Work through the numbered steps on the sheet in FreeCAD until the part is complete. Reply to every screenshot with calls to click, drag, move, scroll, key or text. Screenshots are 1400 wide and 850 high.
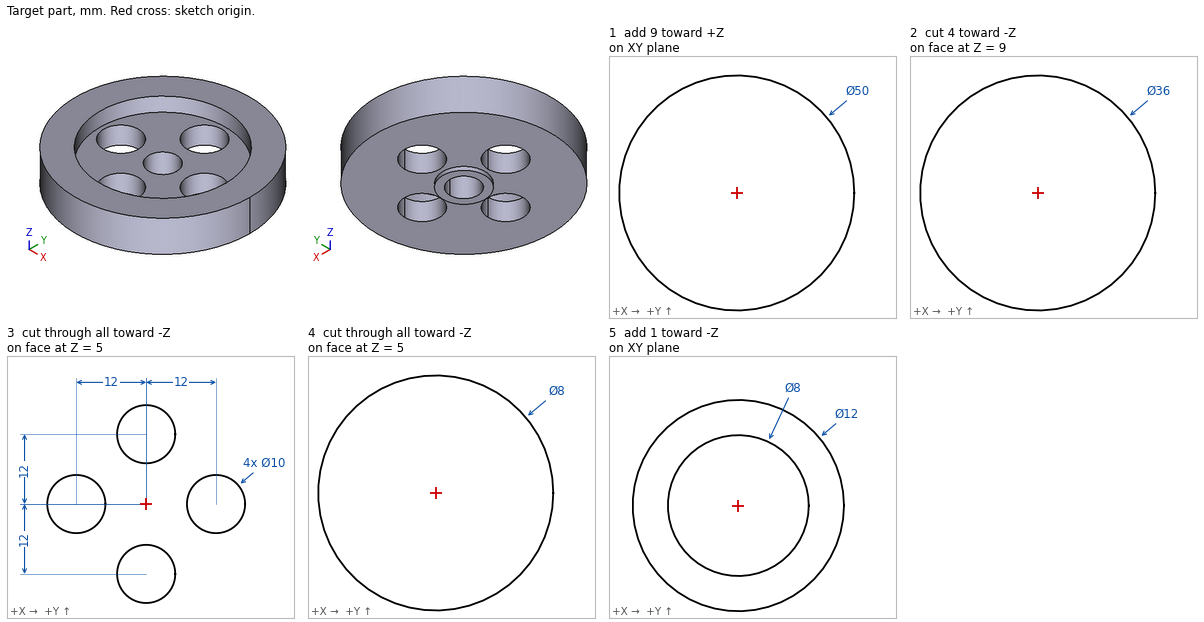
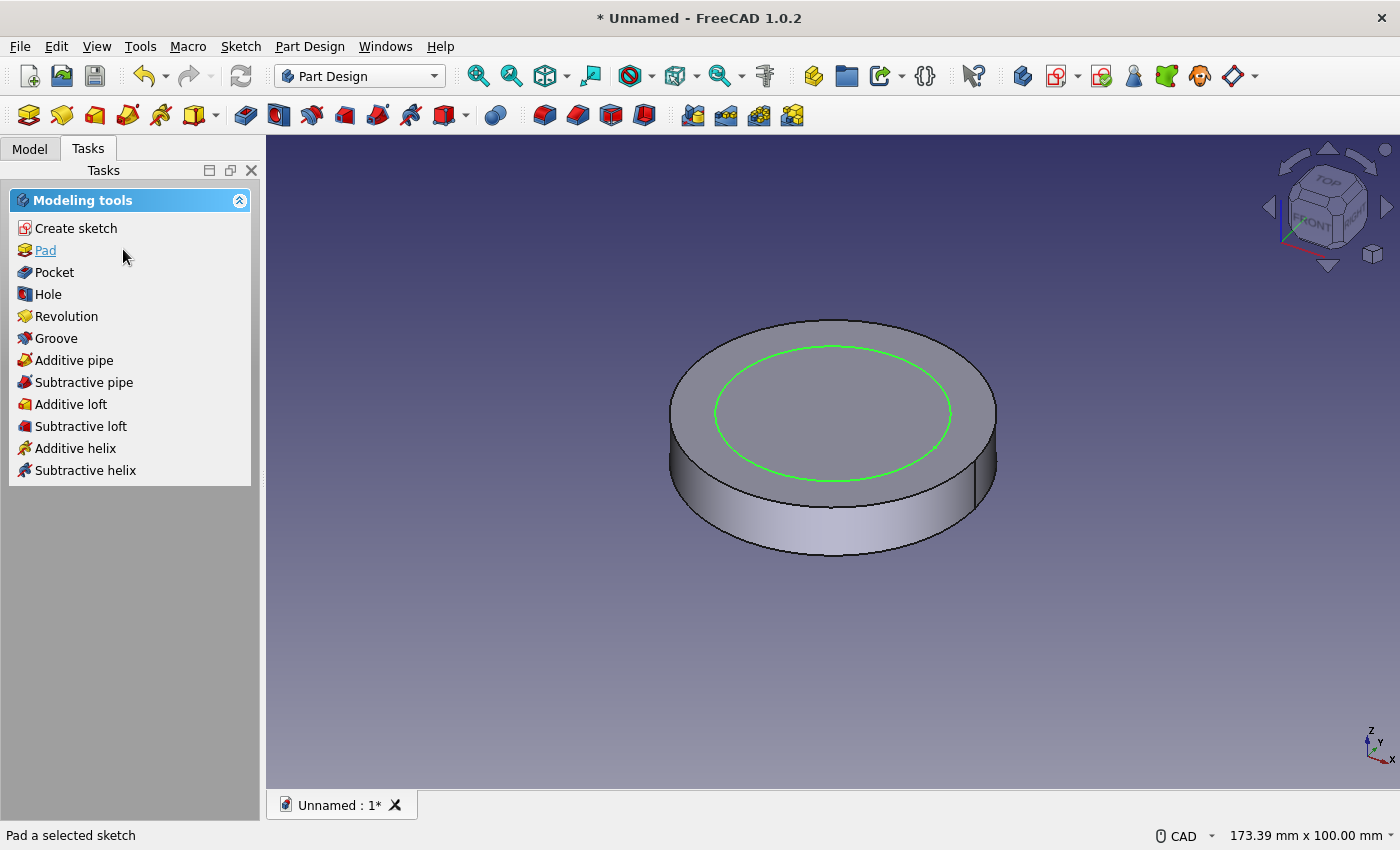
click(246, 116)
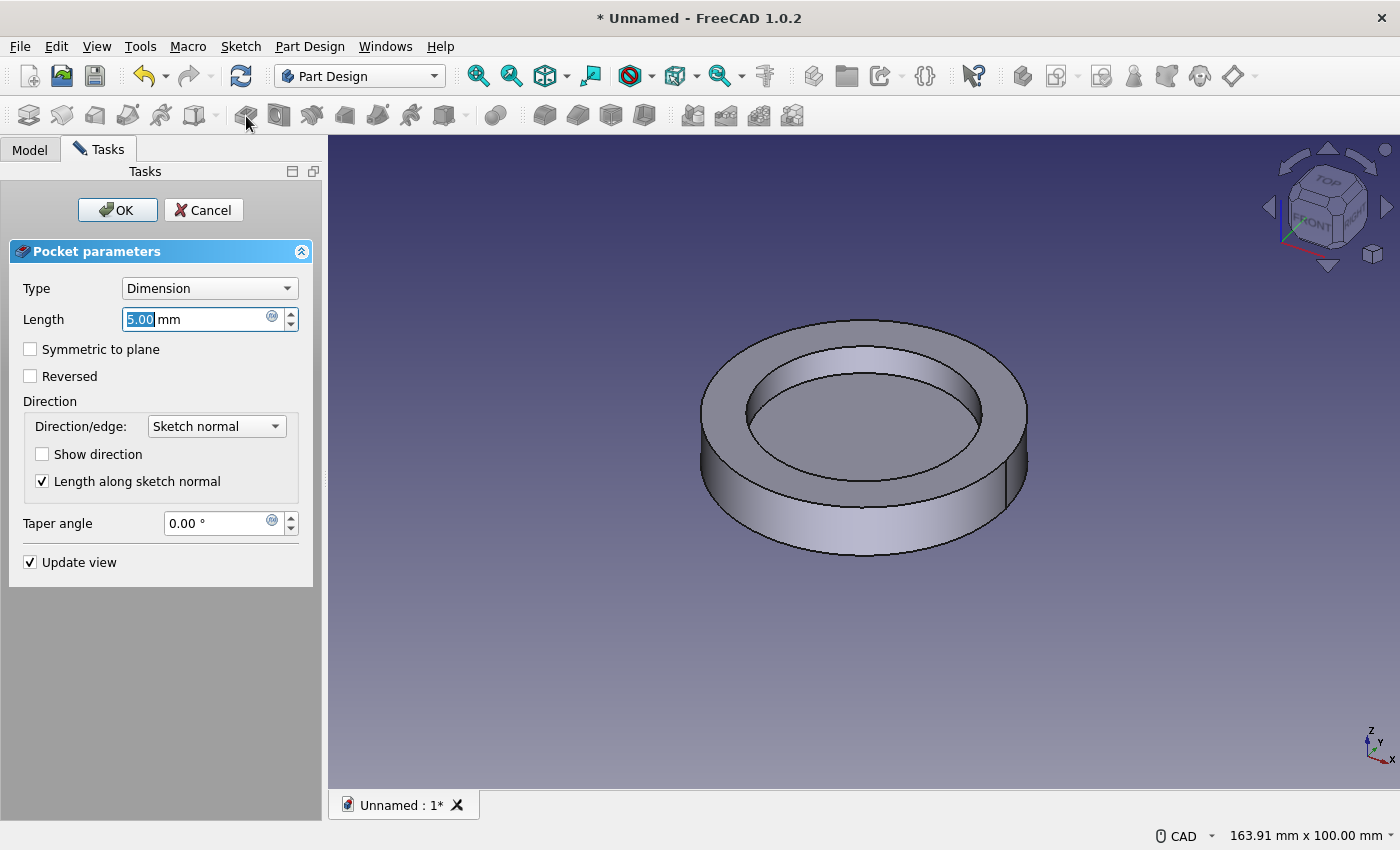
text(4)
key(Tab)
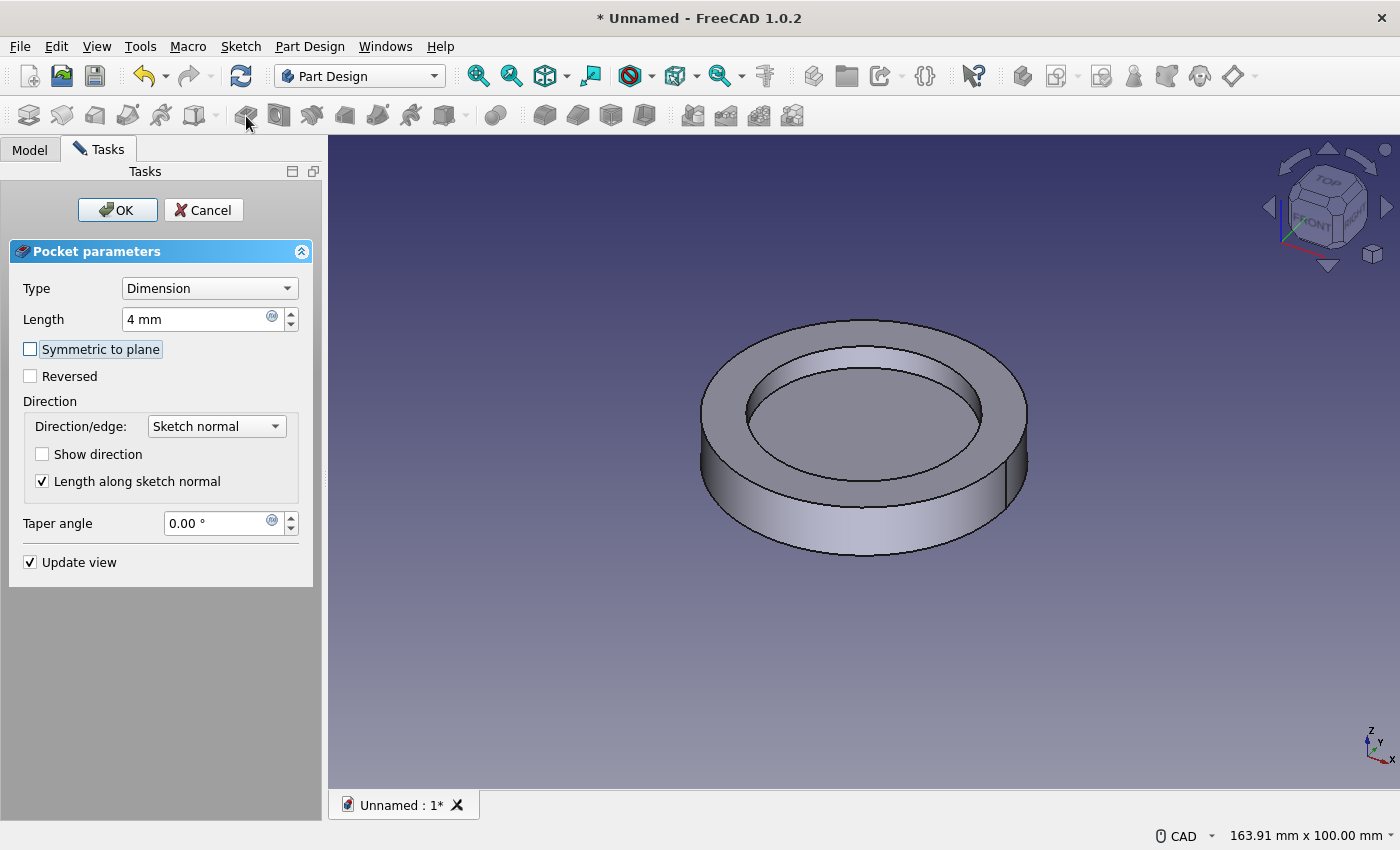
click(118, 210)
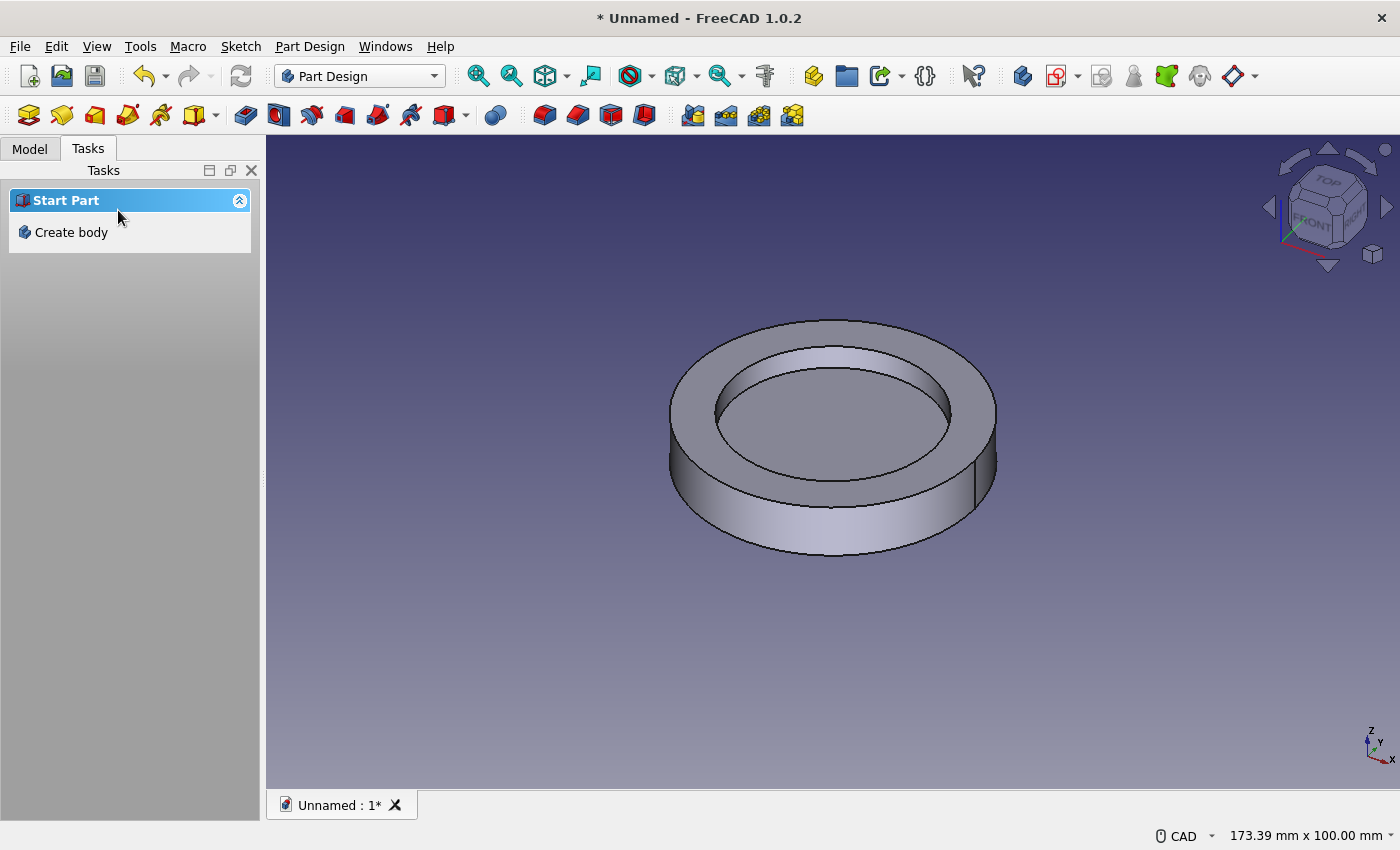
click(833, 434)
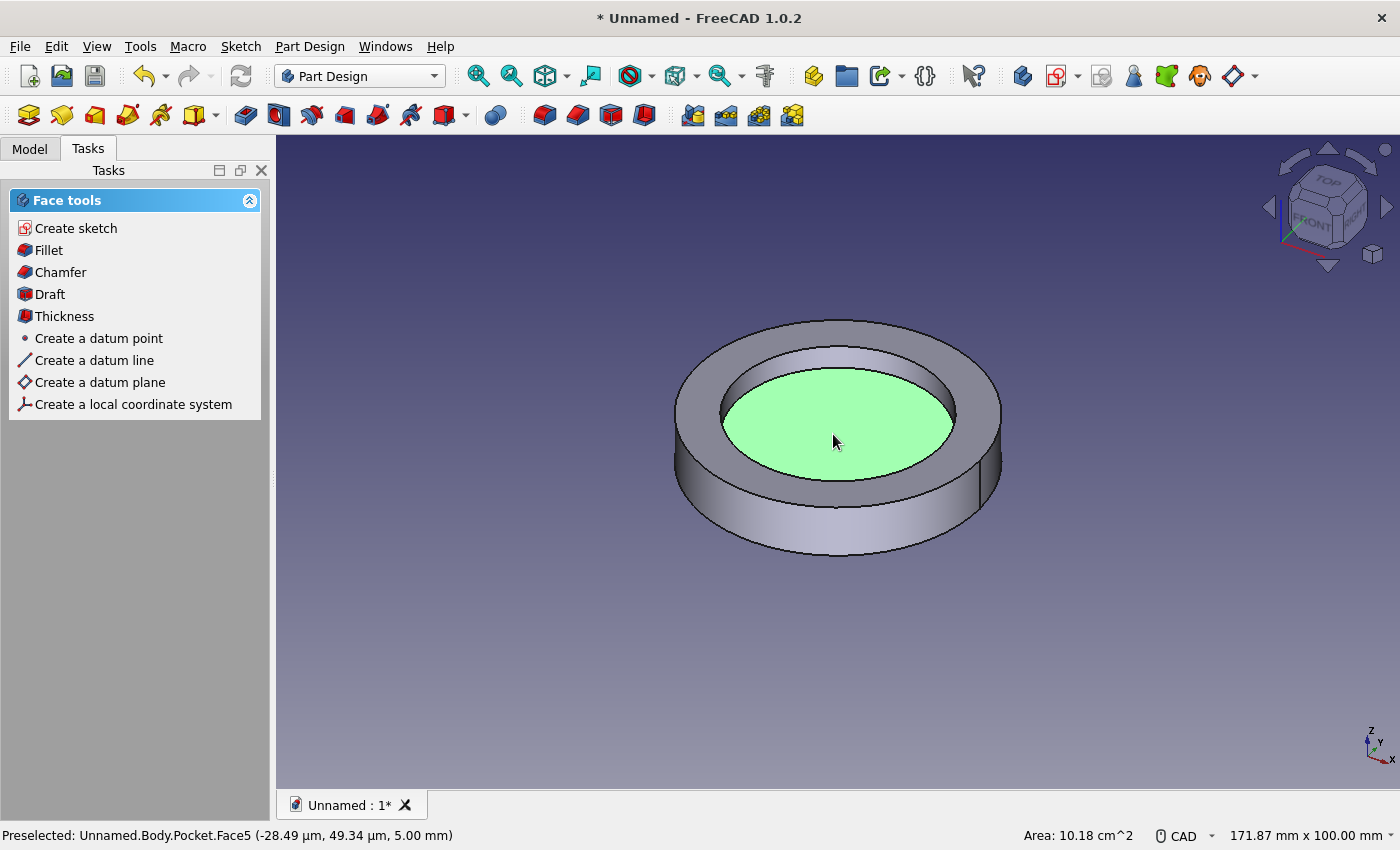
click(1056, 76)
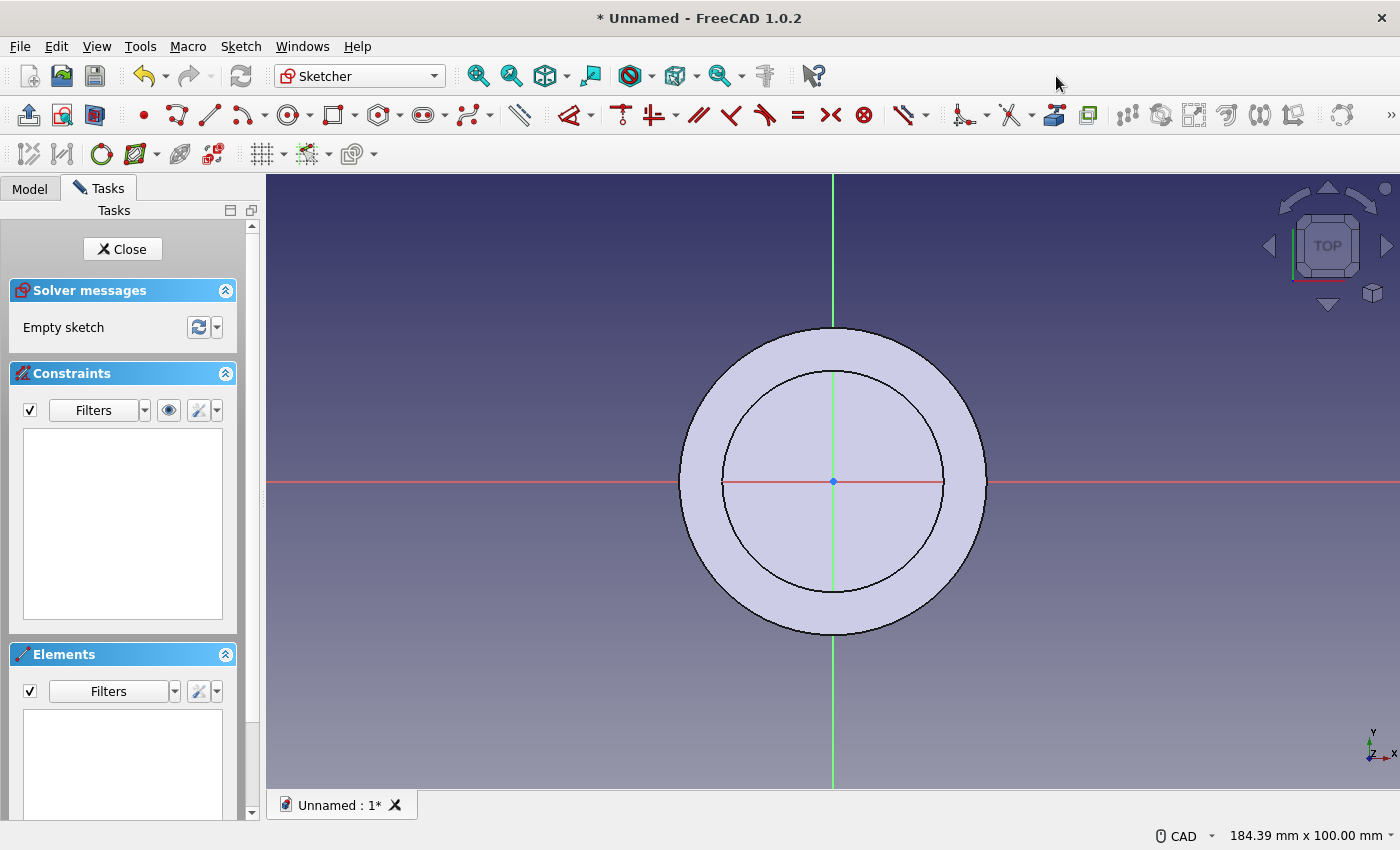
click(95, 116)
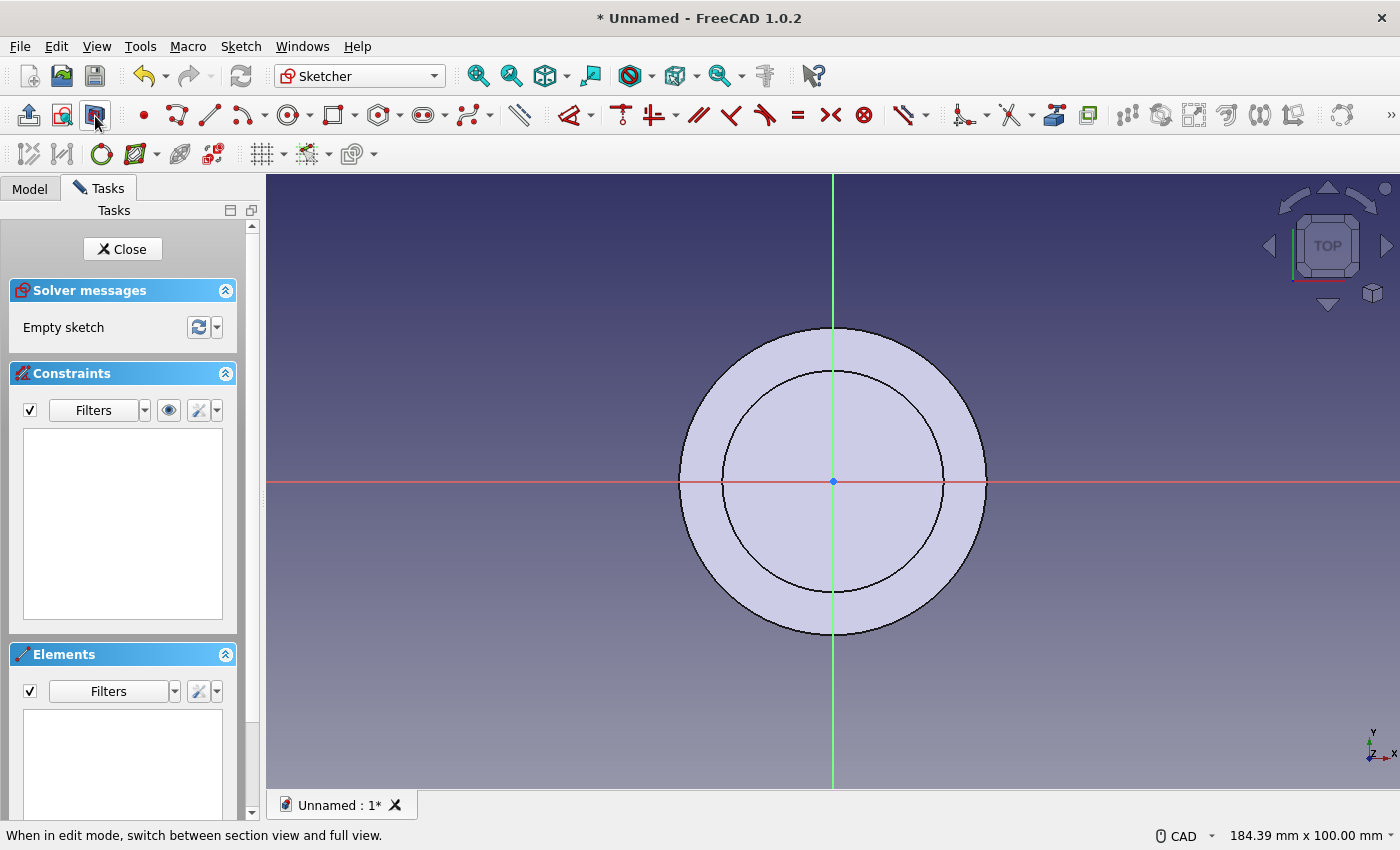
scroll(916, 481, up, 3)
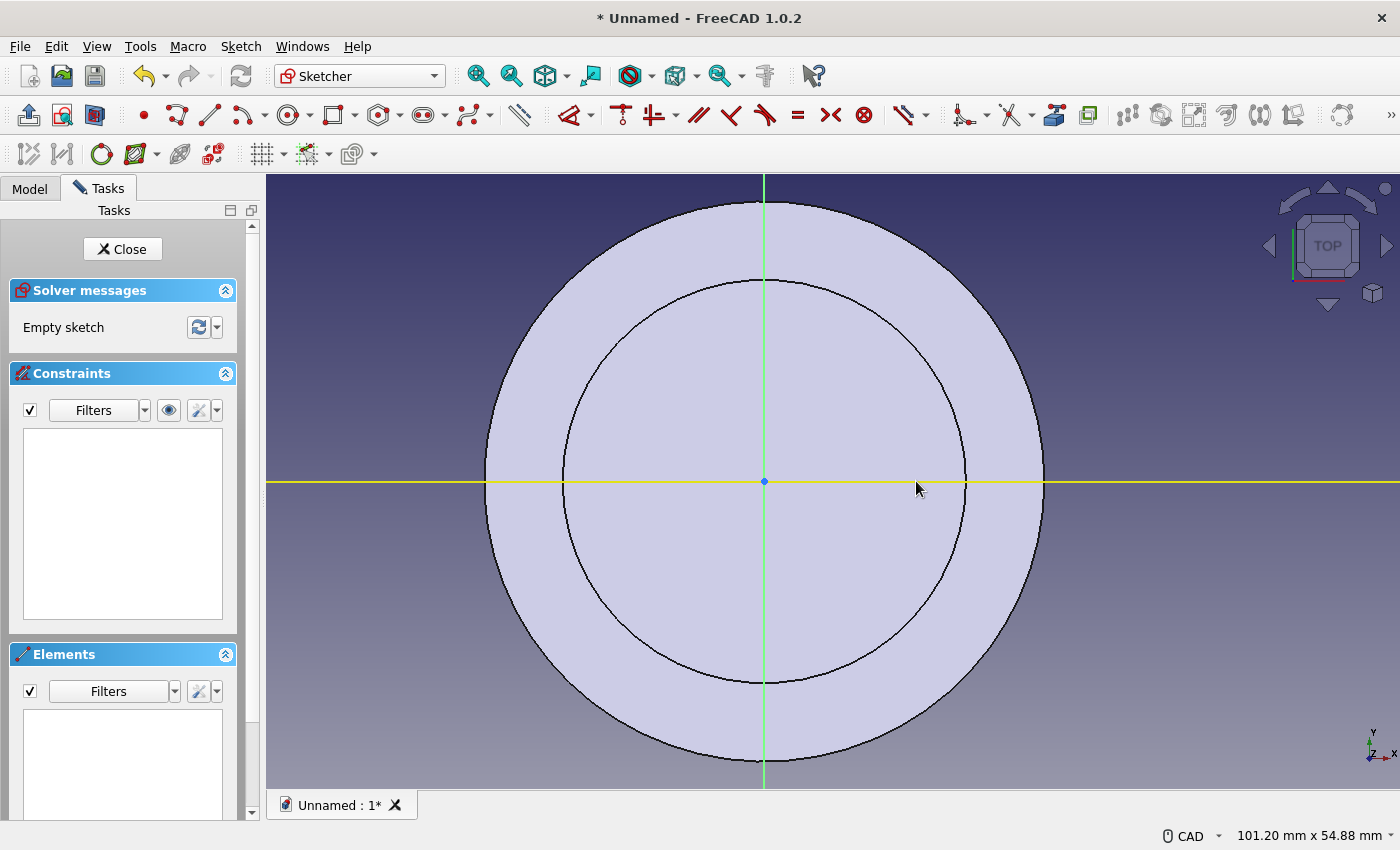
click(288, 116)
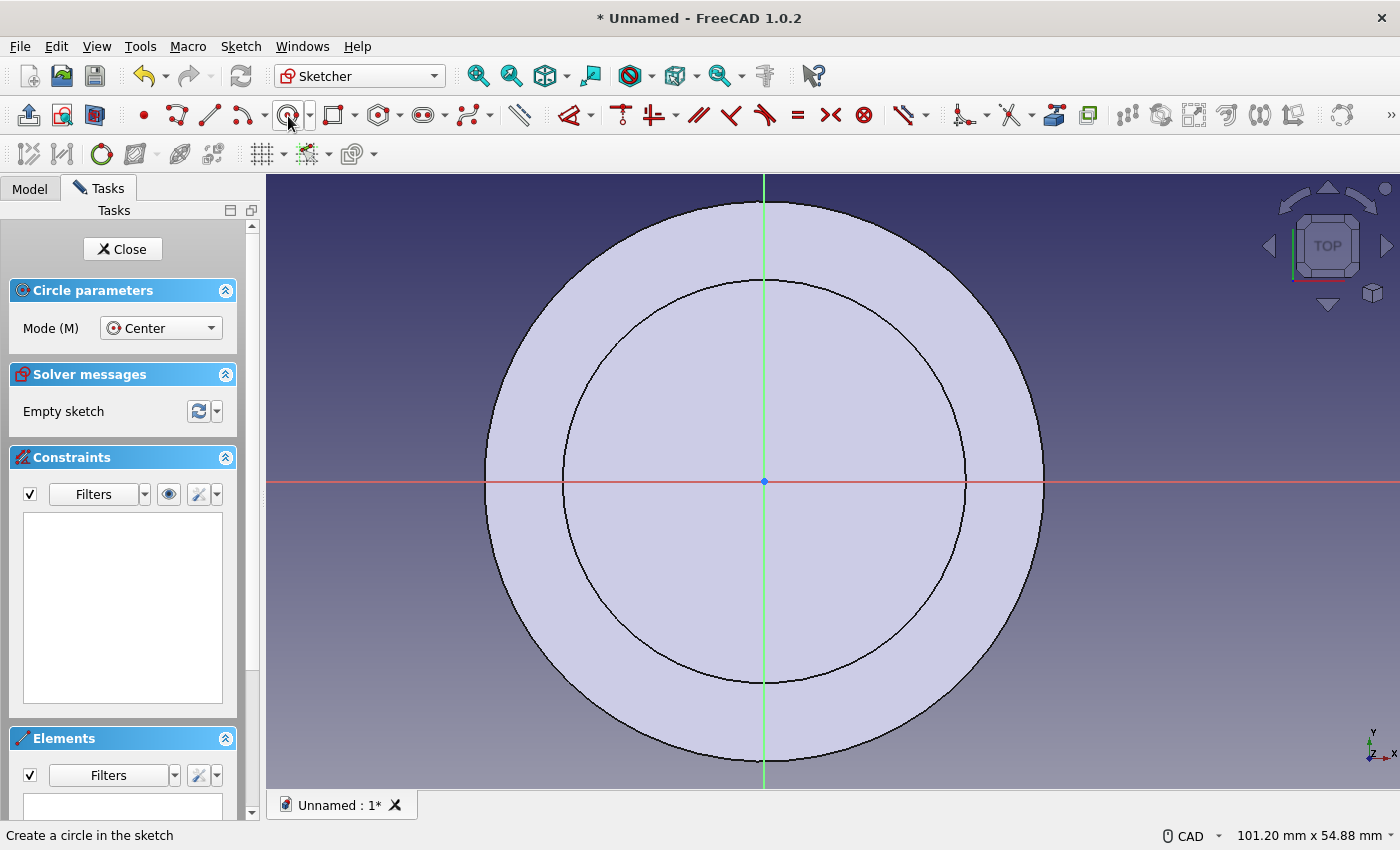
click(764, 347)
move(804, 307)